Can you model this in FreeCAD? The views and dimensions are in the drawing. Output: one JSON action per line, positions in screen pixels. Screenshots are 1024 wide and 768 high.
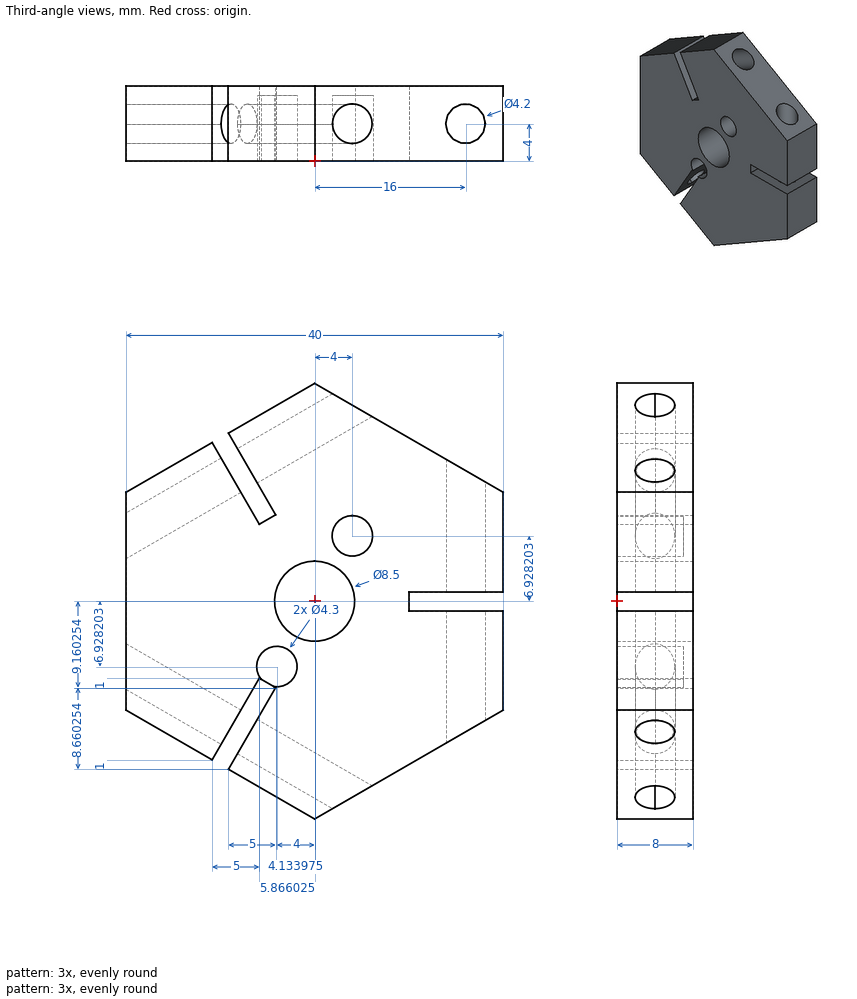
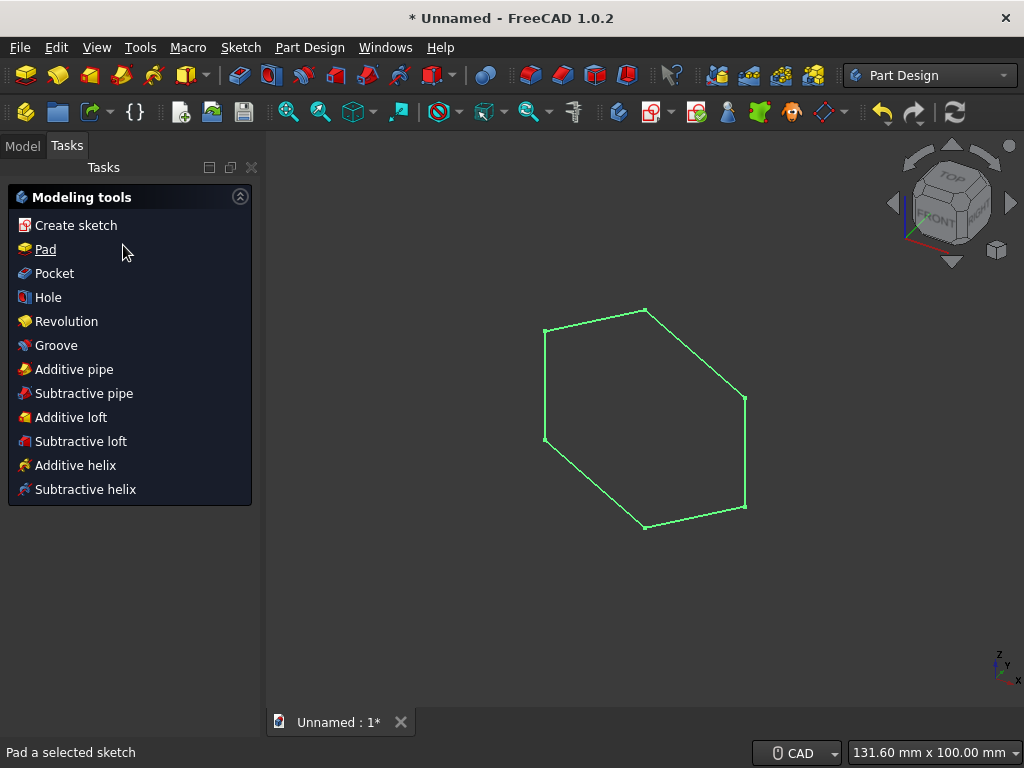
{"action": "left_click", "coordinate": [26, 76]}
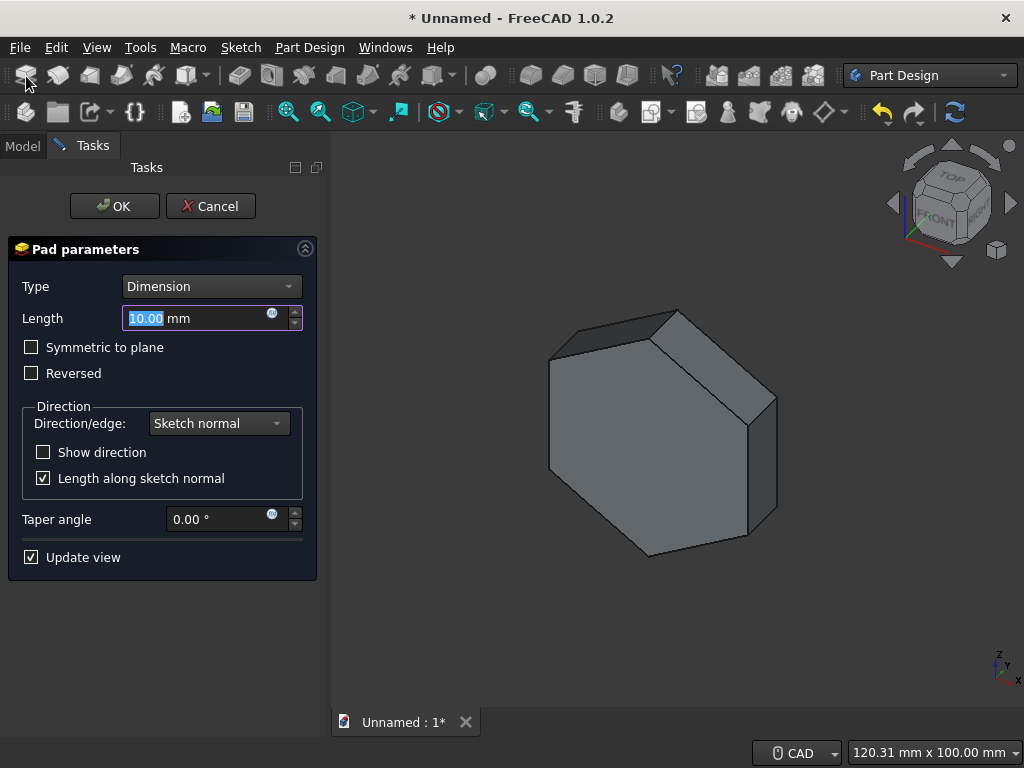
{"action": "type", "text": "8"}
{"action": "key", "text": "Tab"}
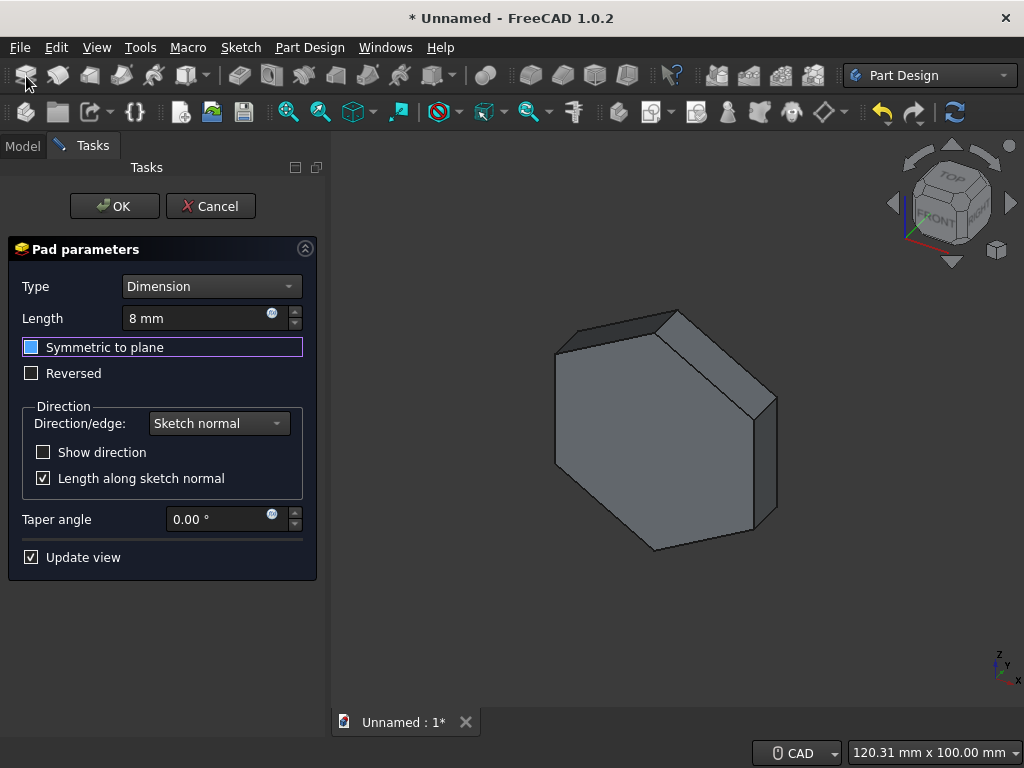
{"action": "left_click", "coordinate": [30, 373]}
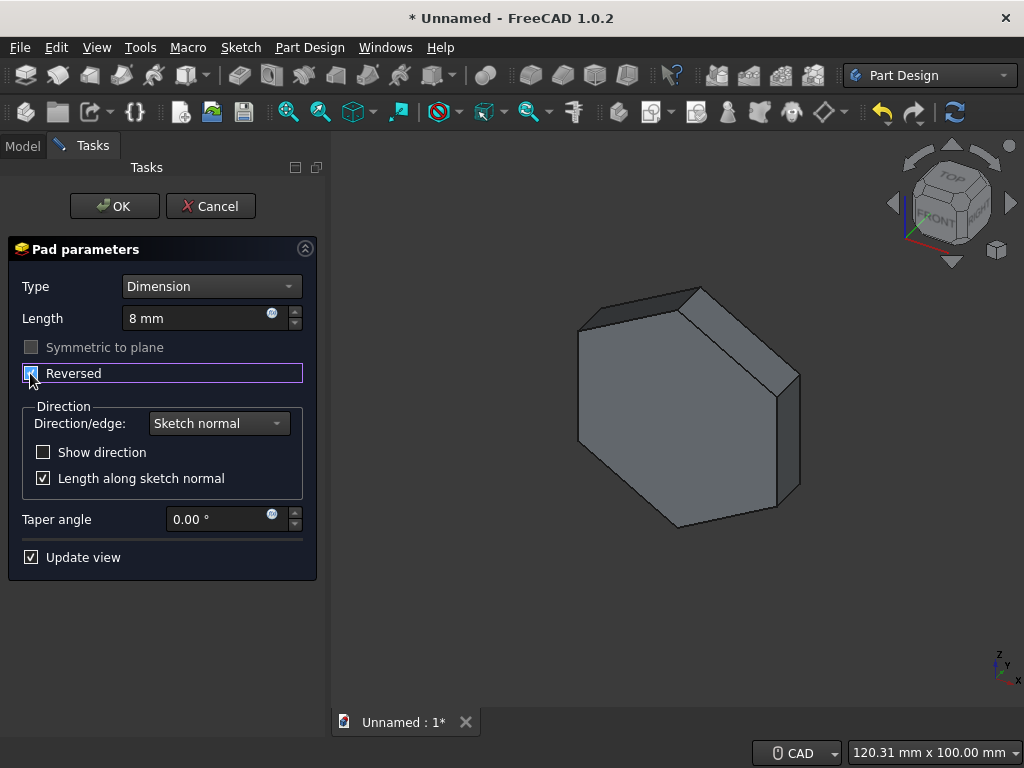
{"action": "left_click", "coordinate": [115, 206]}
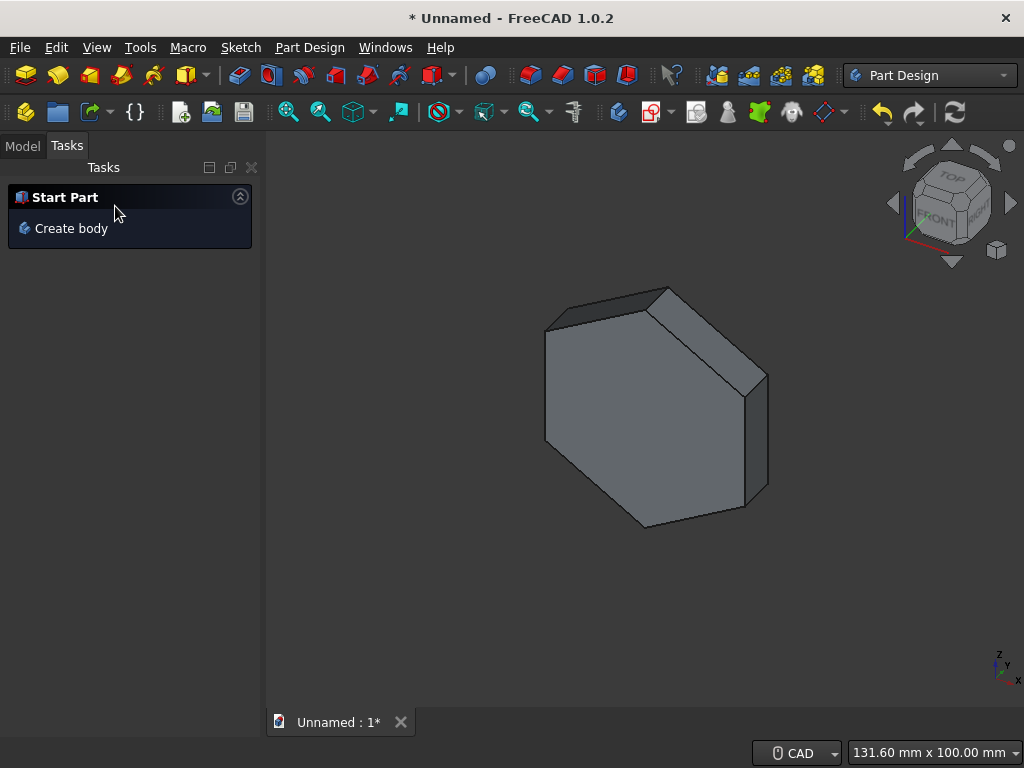
{"action": "key", "text": "4"}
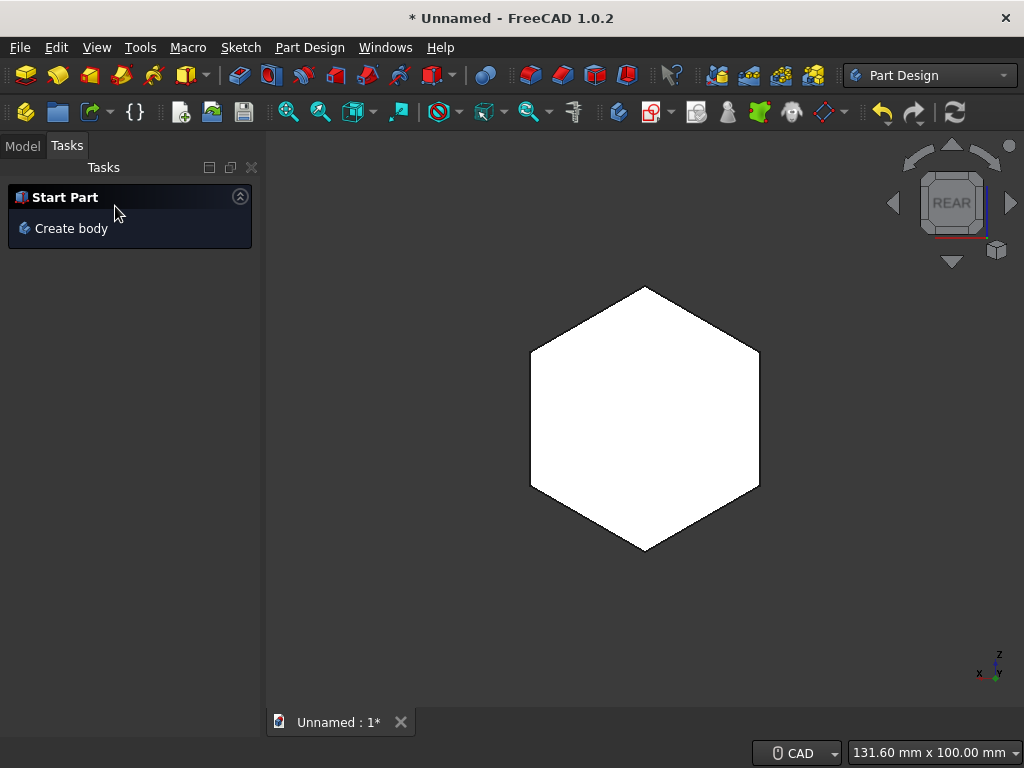
{"action": "left_click", "coordinate": [645, 418]}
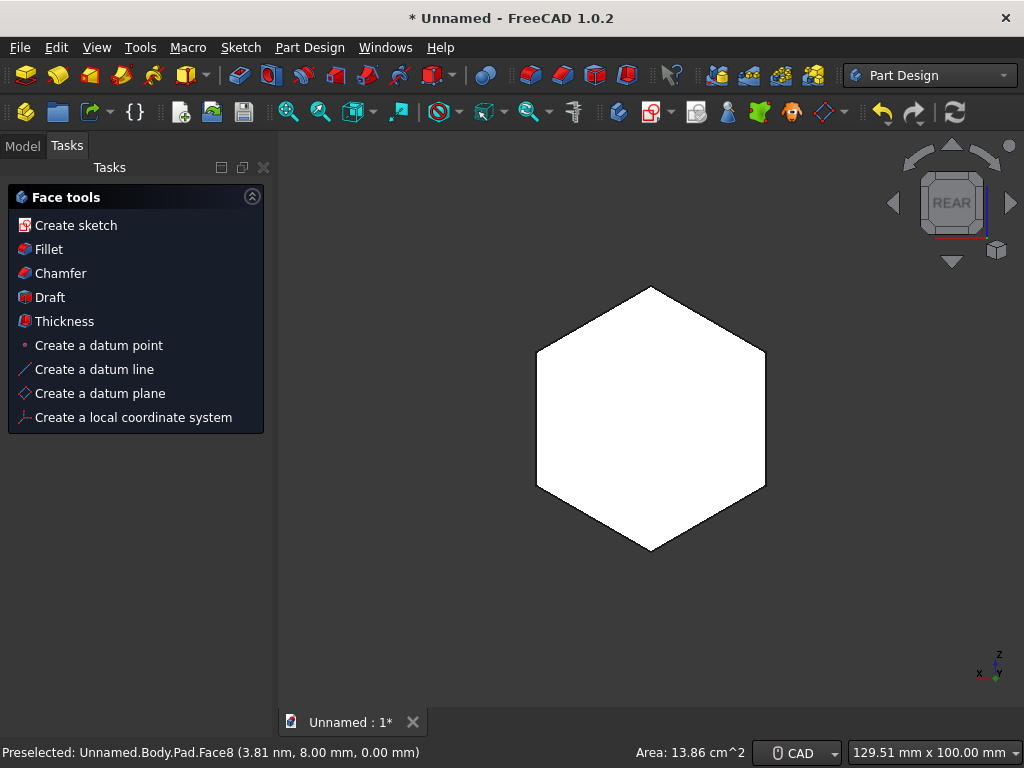
{"action": "left_click", "coordinate": [652, 112]}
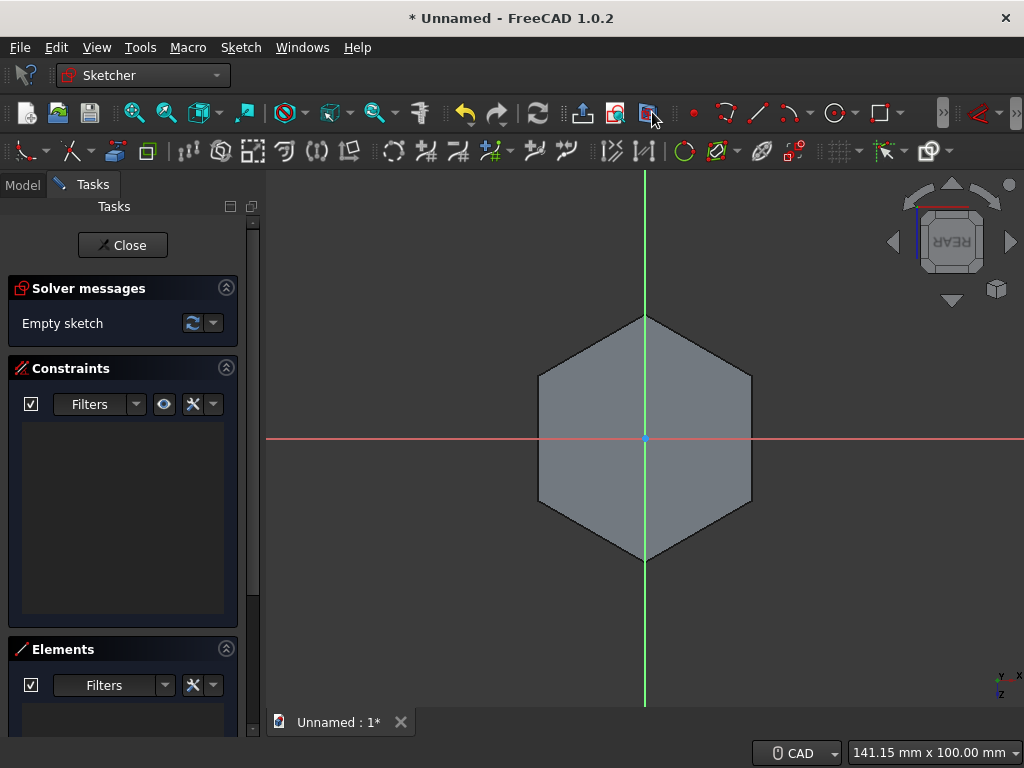
{"action": "scroll", "coordinate": [656, 439], "scroll_direction": "up", "scroll_amount": 10}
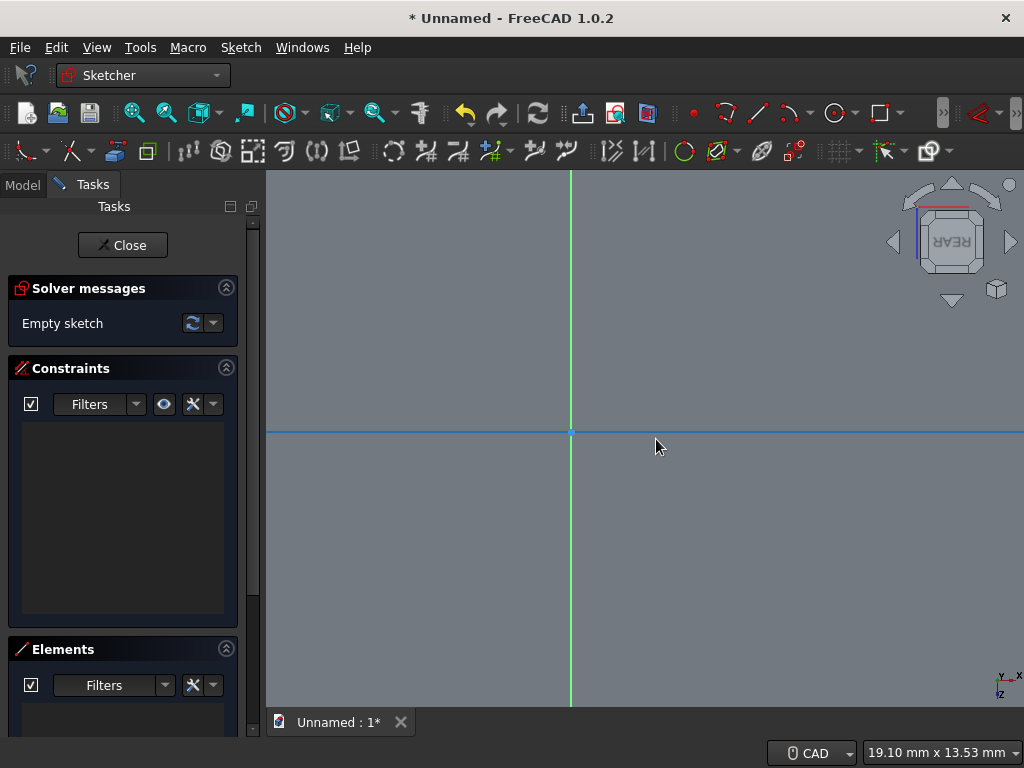
{"action": "left_click", "coordinate": [836, 114]}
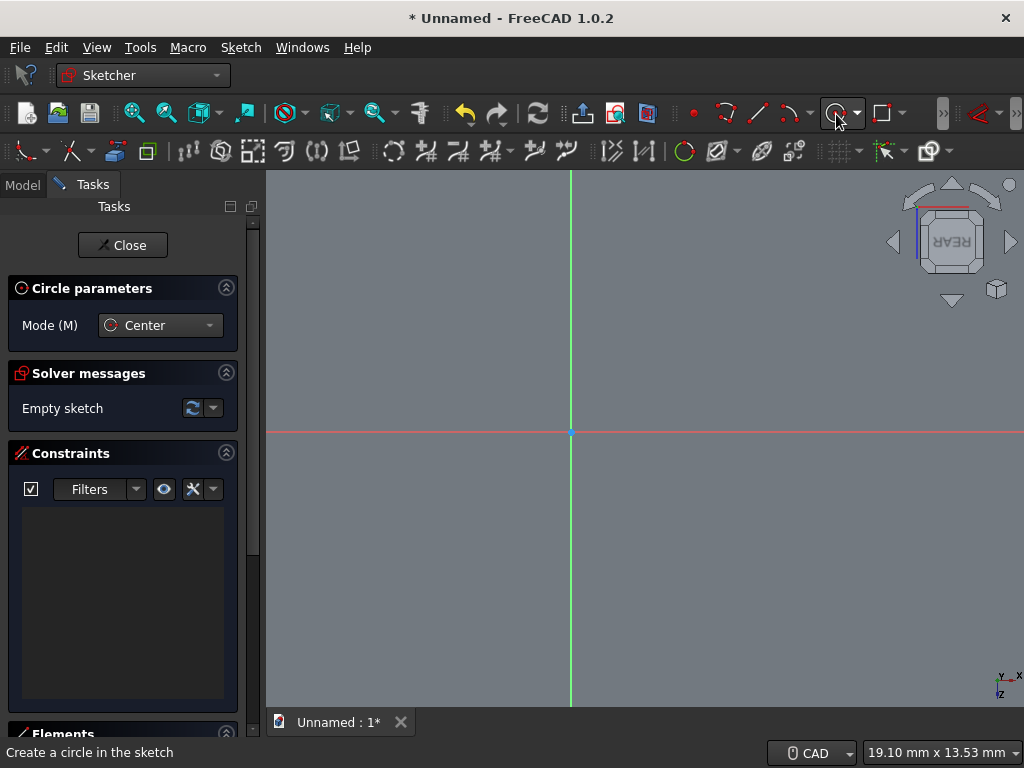
{"action": "left_click", "coordinate": [571, 432]}
{"action": "mouse_move", "coordinate": [691, 313]}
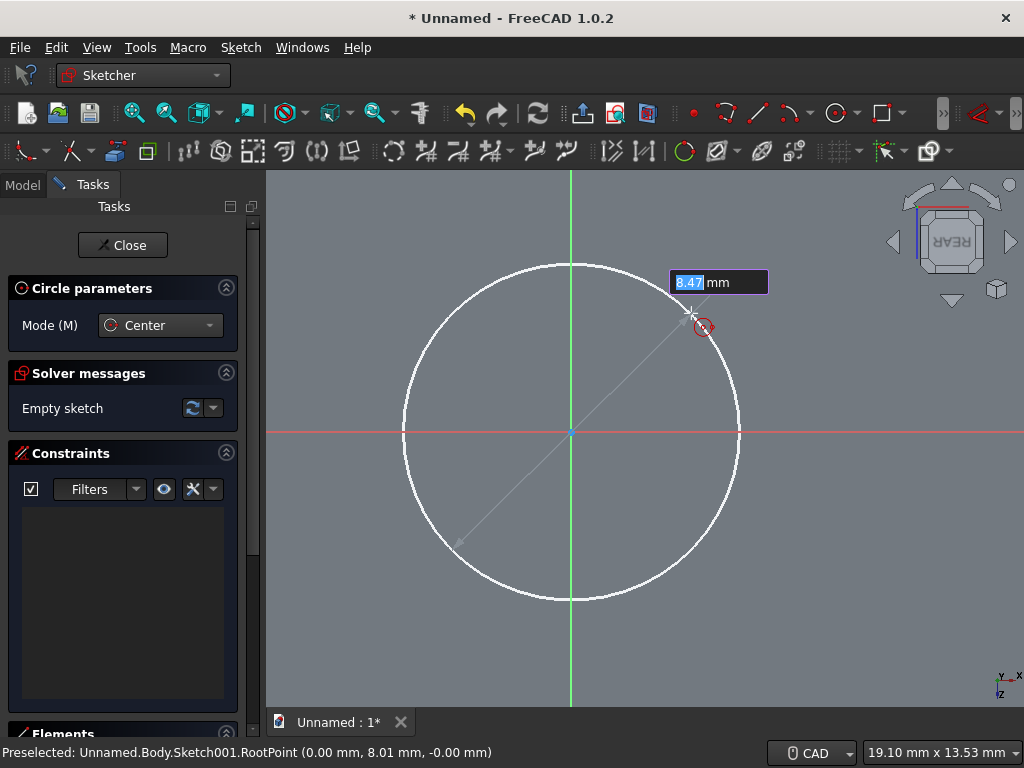
{"action": "type", "text": "8.5"}
{"action": "key", "text": "Return"}
{"action": "key", "text": "Escape"}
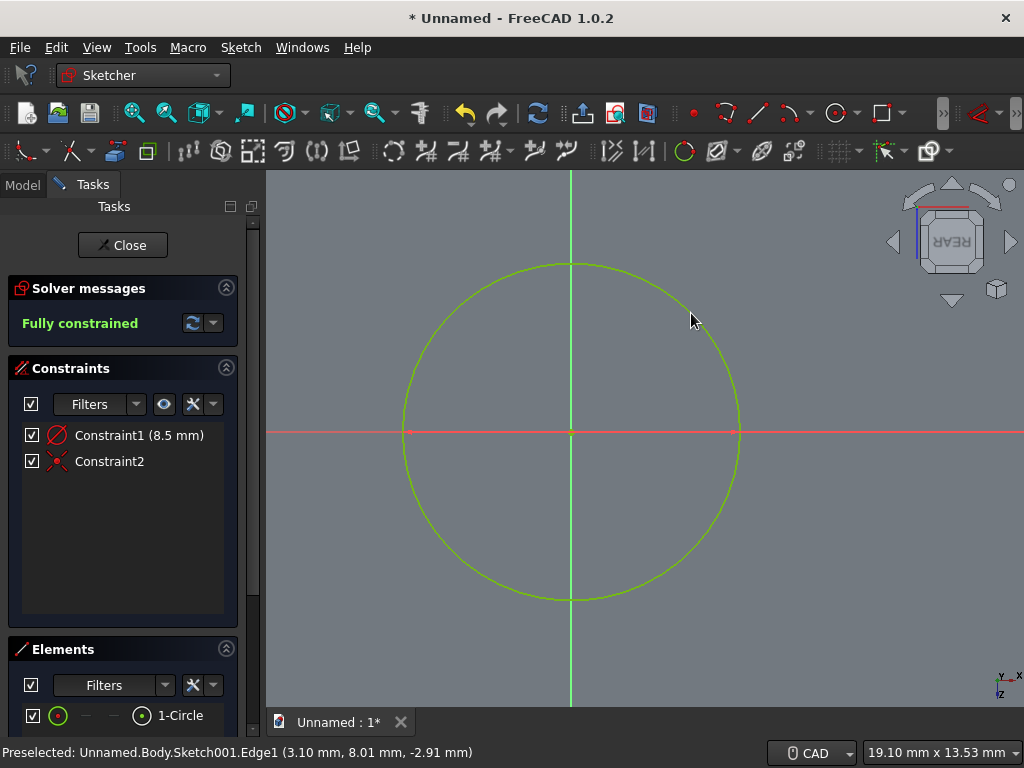
{"action": "left_click", "coordinate": [123, 245]}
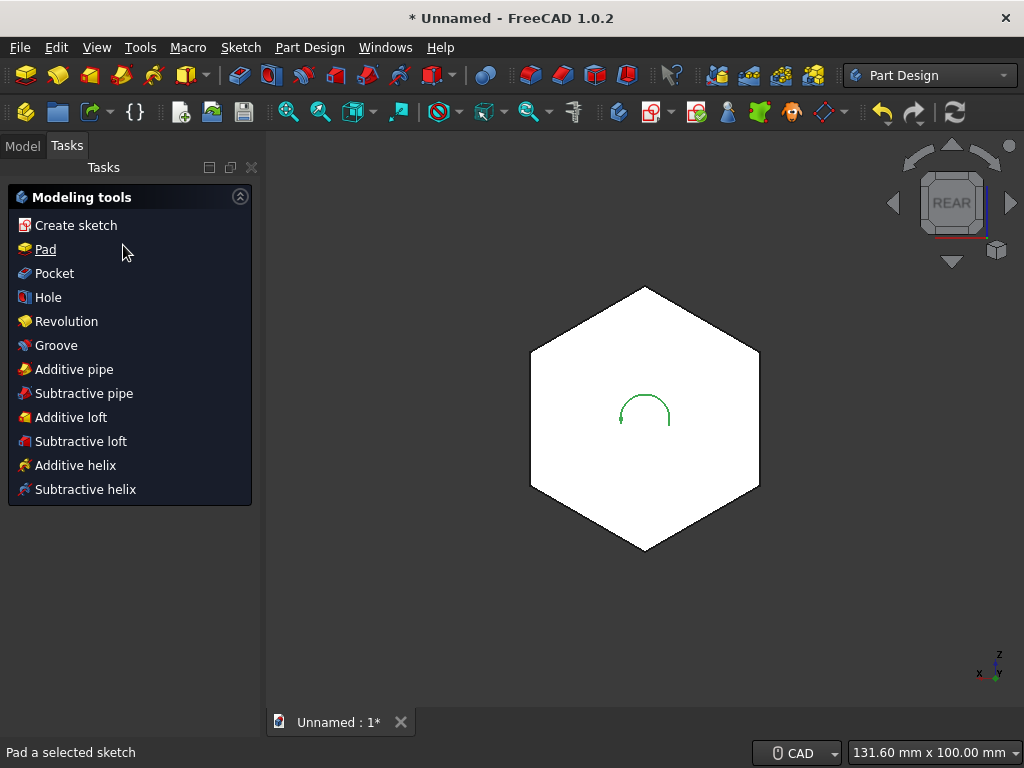
{"action": "left_click", "coordinate": [240, 76]}